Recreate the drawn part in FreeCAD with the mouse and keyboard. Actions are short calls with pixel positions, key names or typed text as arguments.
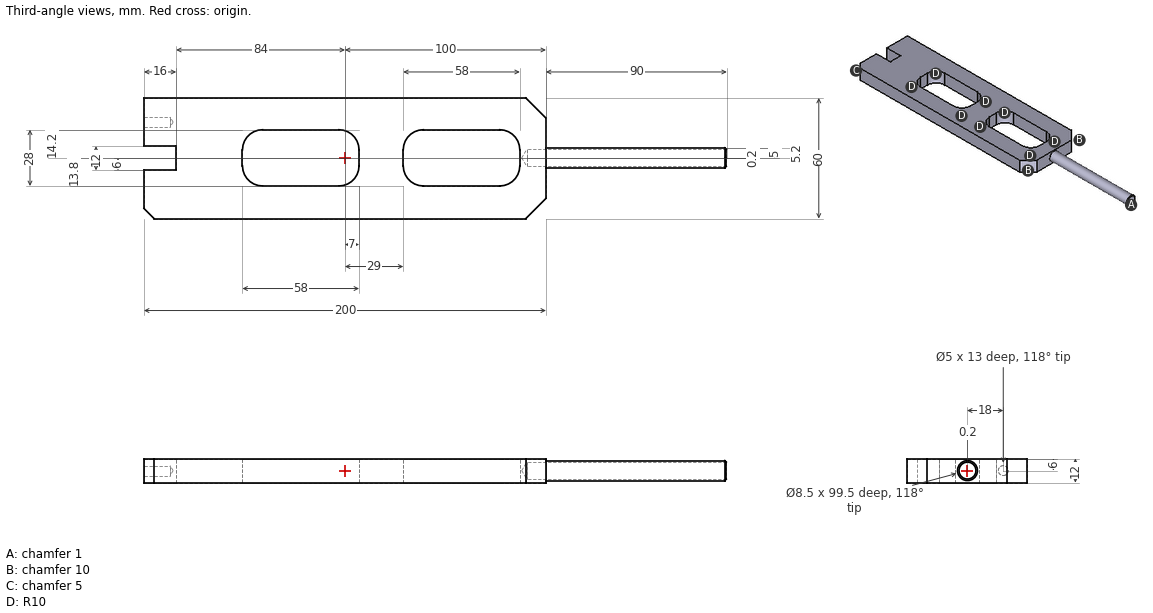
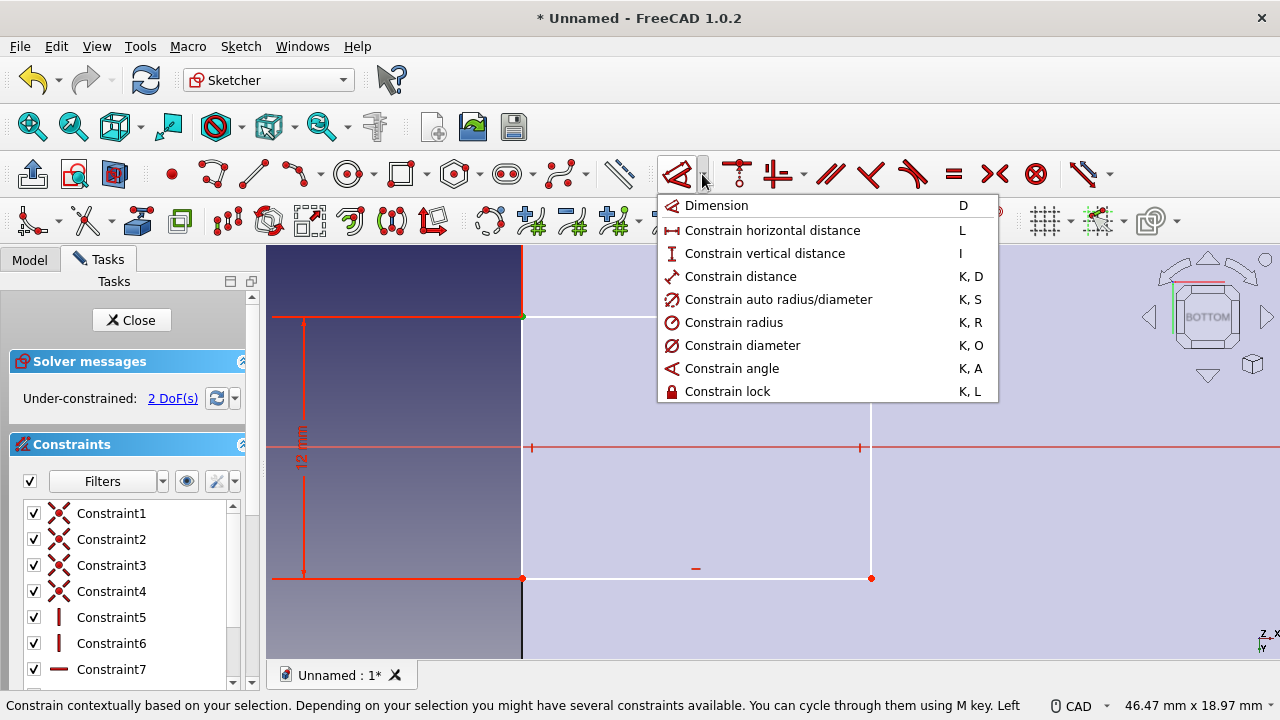
click(828, 254)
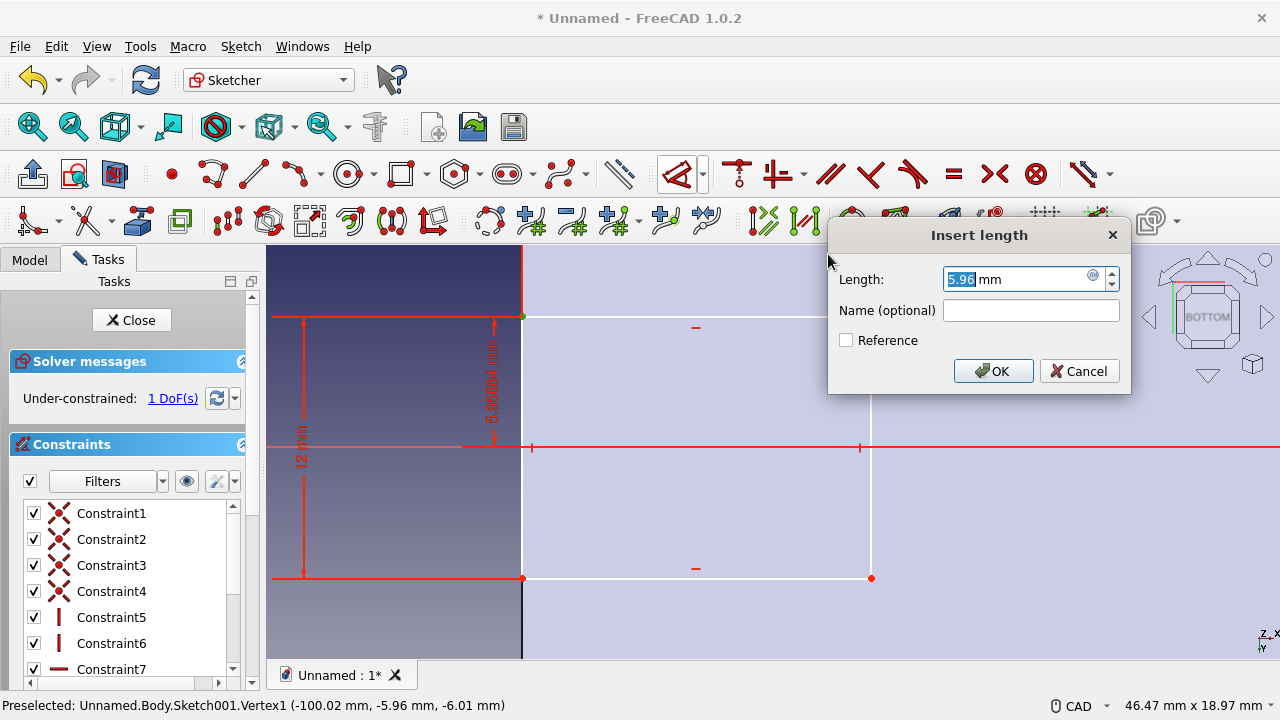
text(6)
key(Return)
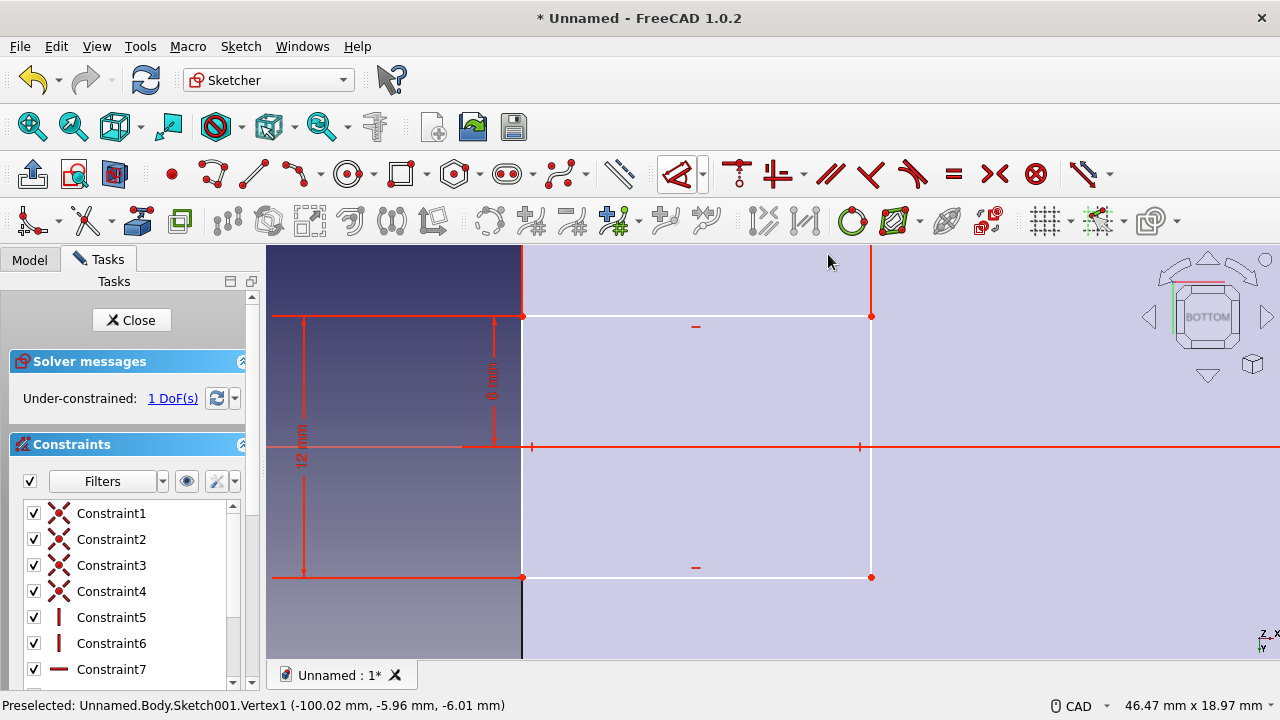
click(871, 578)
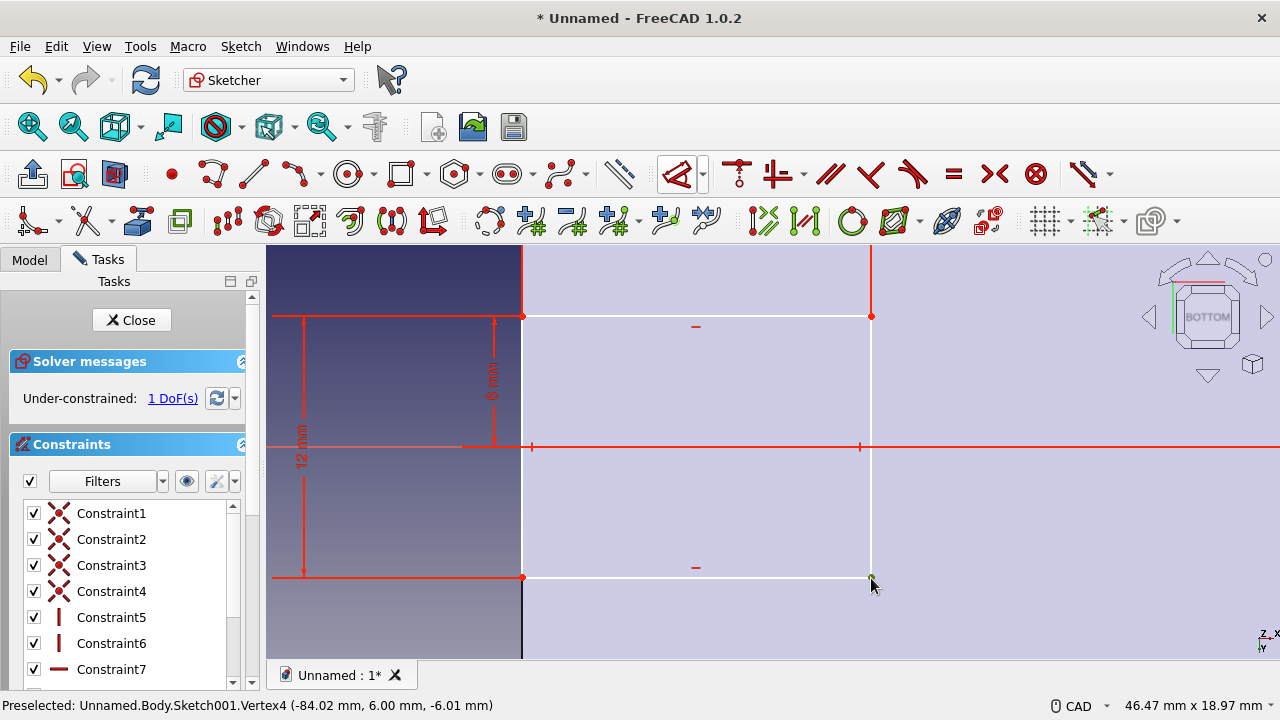
key(l)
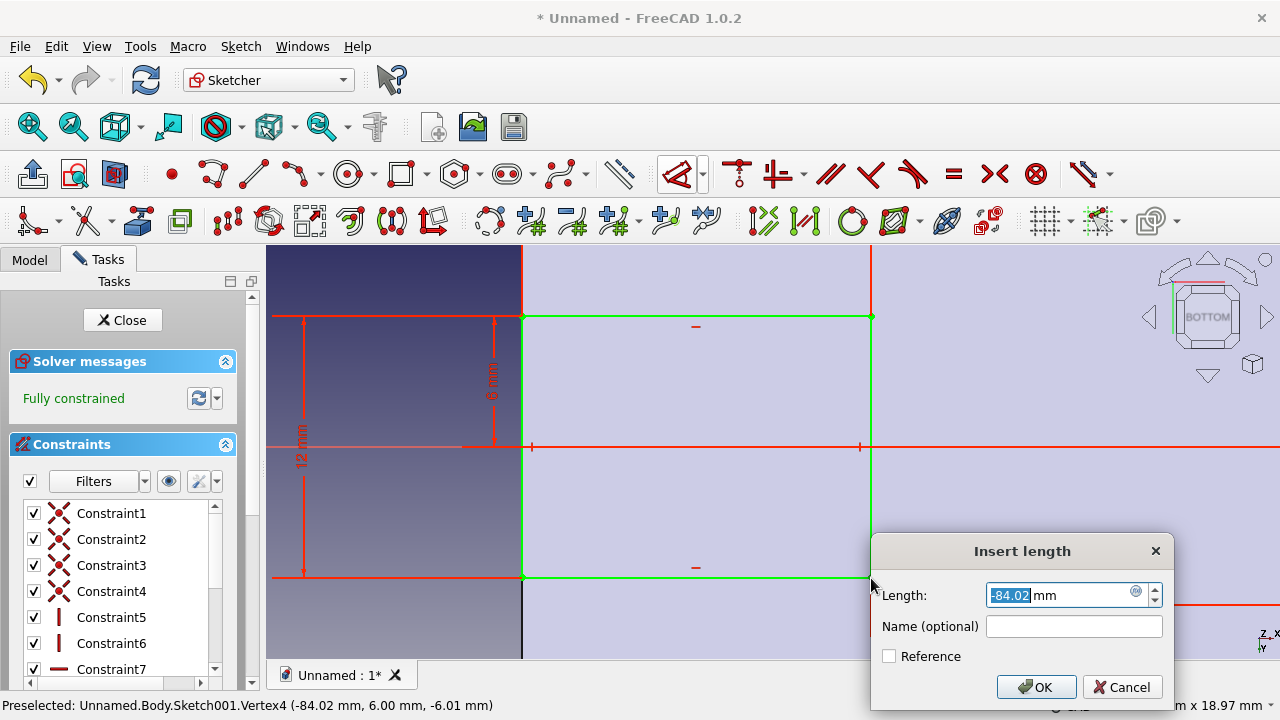
text(-84)
key(Return)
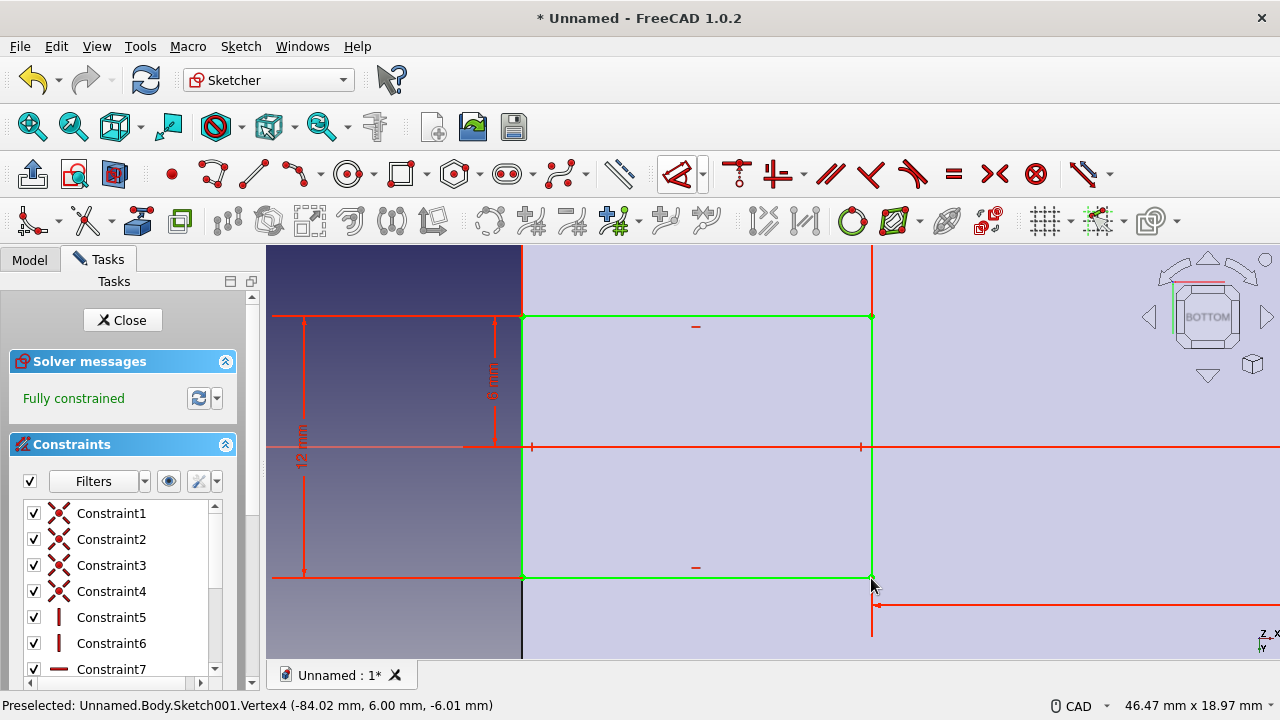
click(123, 320)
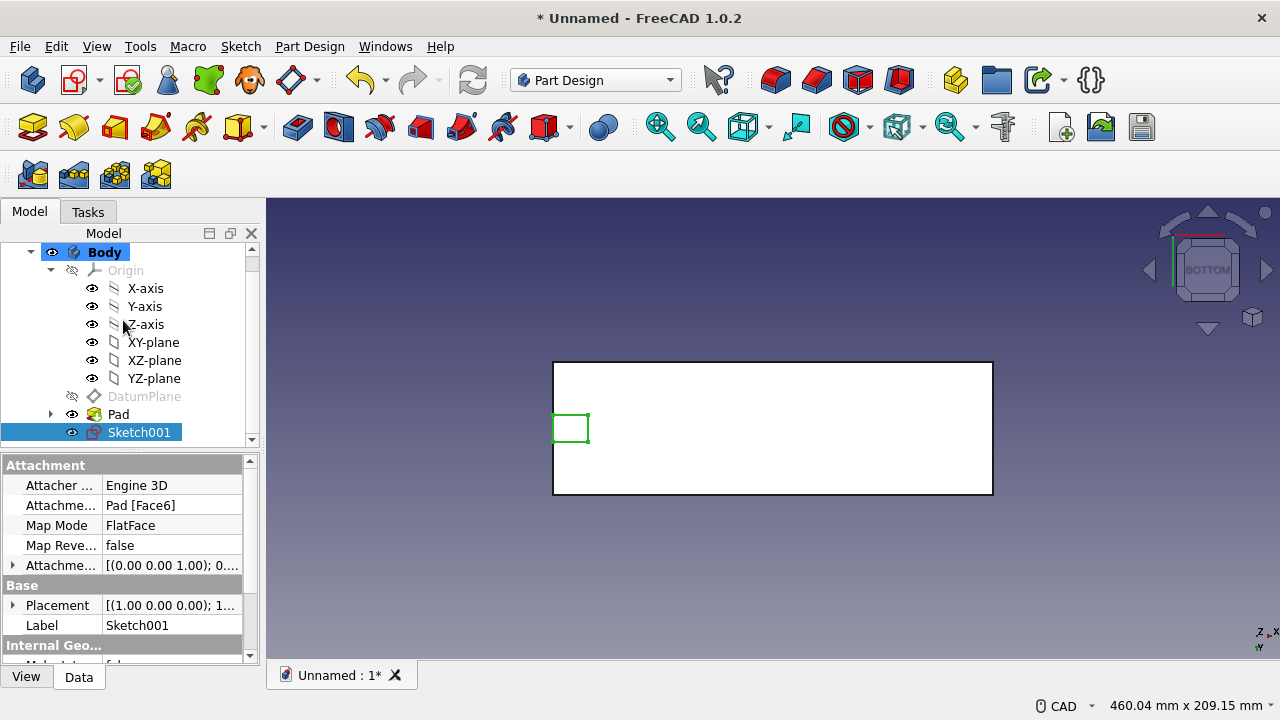
click(298, 128)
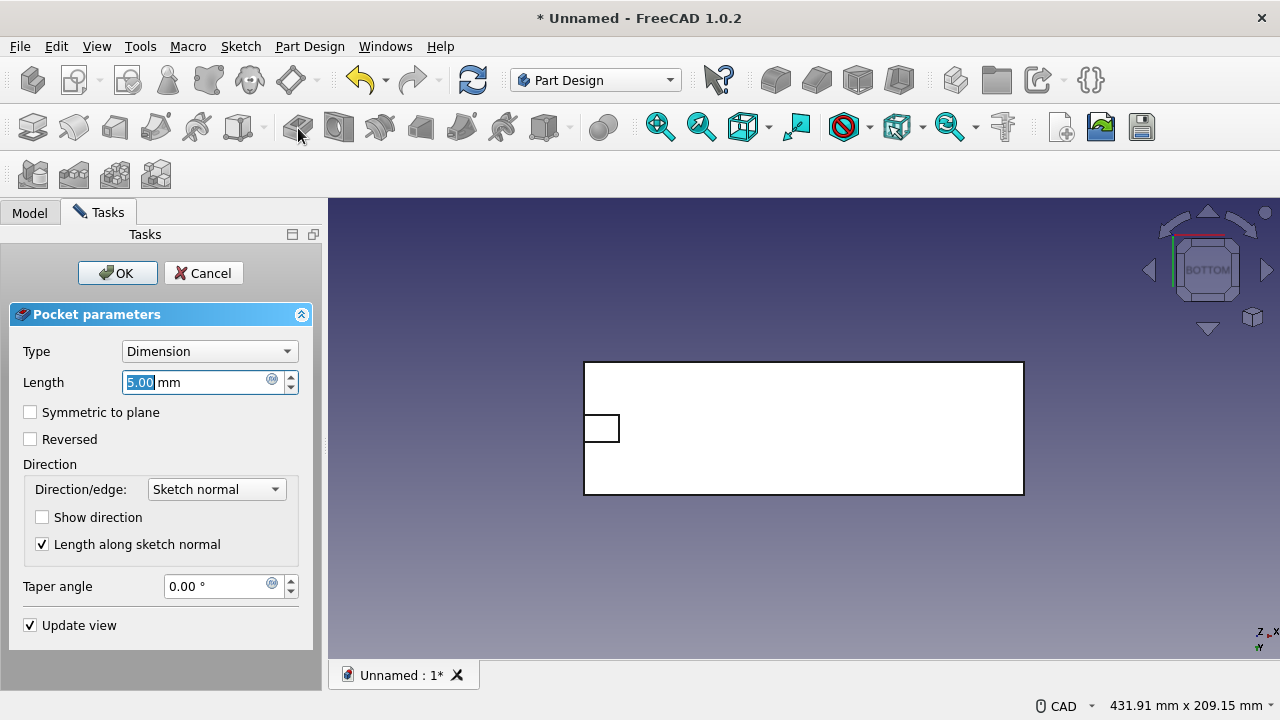
click(210, 352)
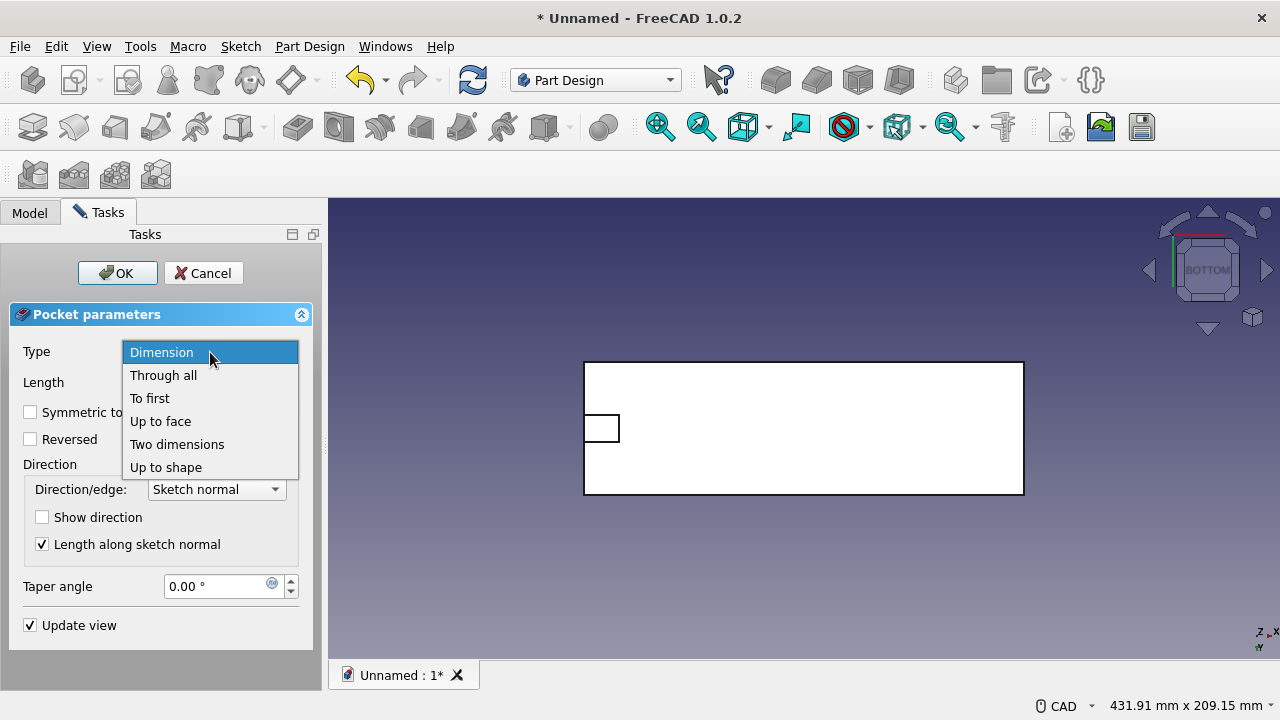
click(208, 376)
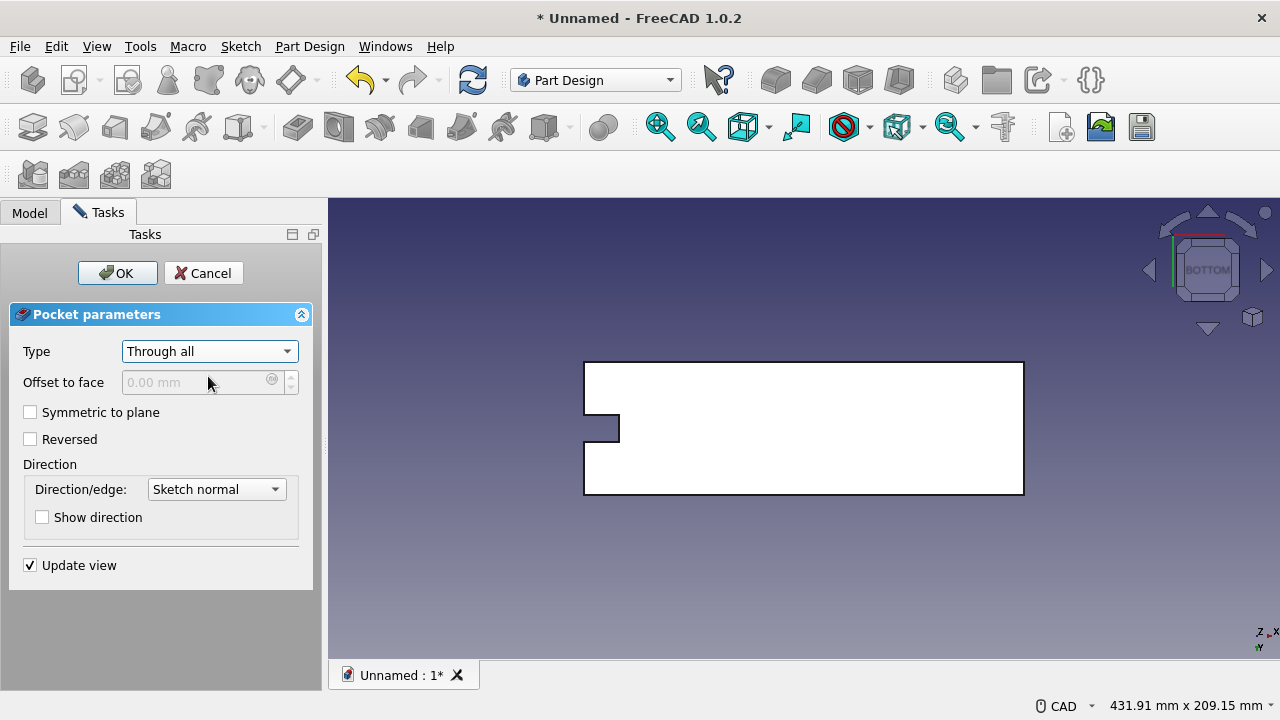
click(118, 273)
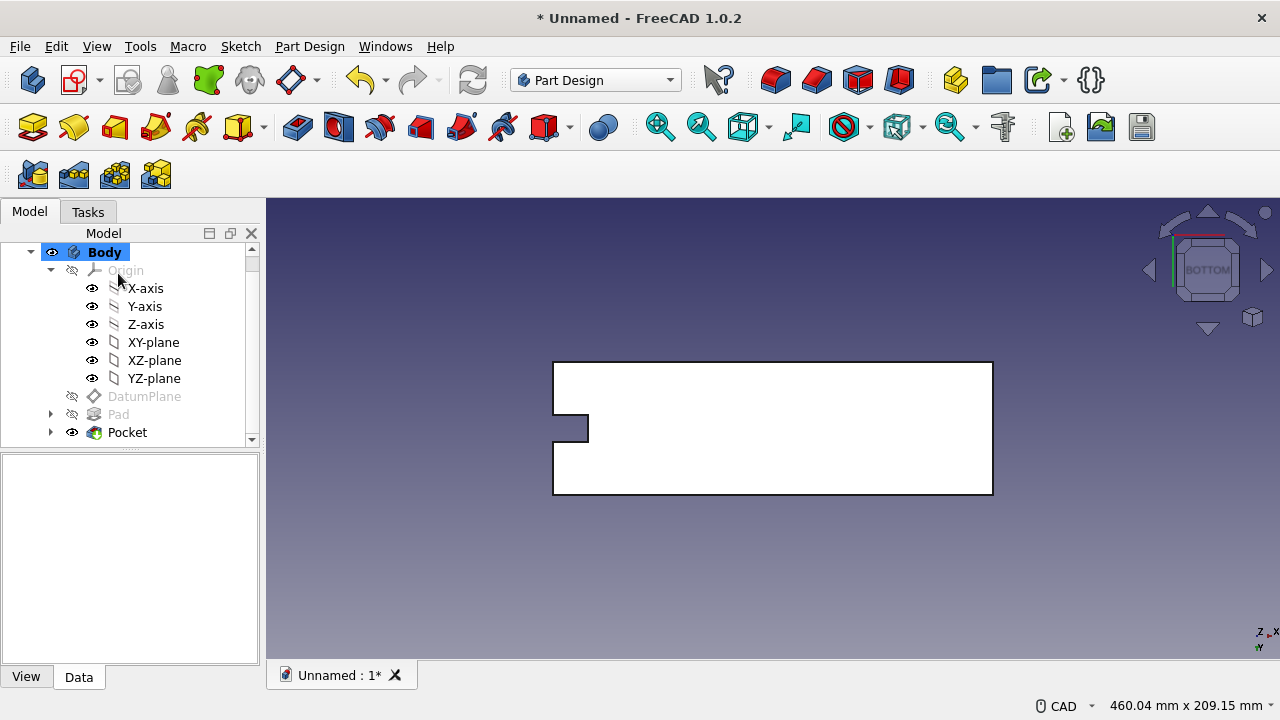
click(661, 128)